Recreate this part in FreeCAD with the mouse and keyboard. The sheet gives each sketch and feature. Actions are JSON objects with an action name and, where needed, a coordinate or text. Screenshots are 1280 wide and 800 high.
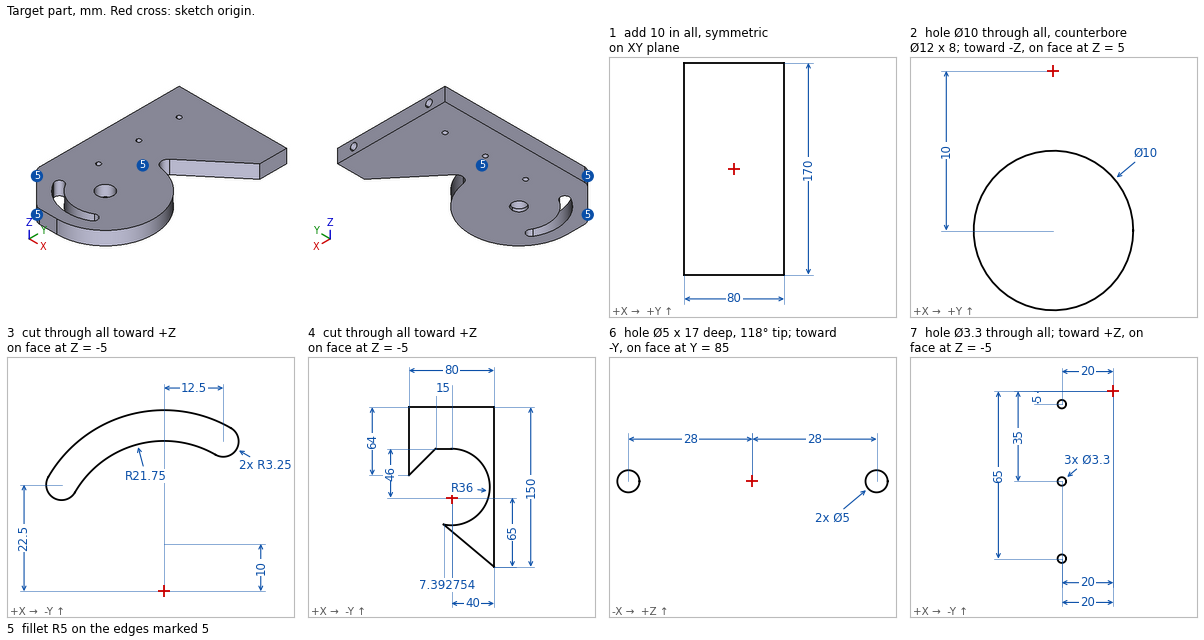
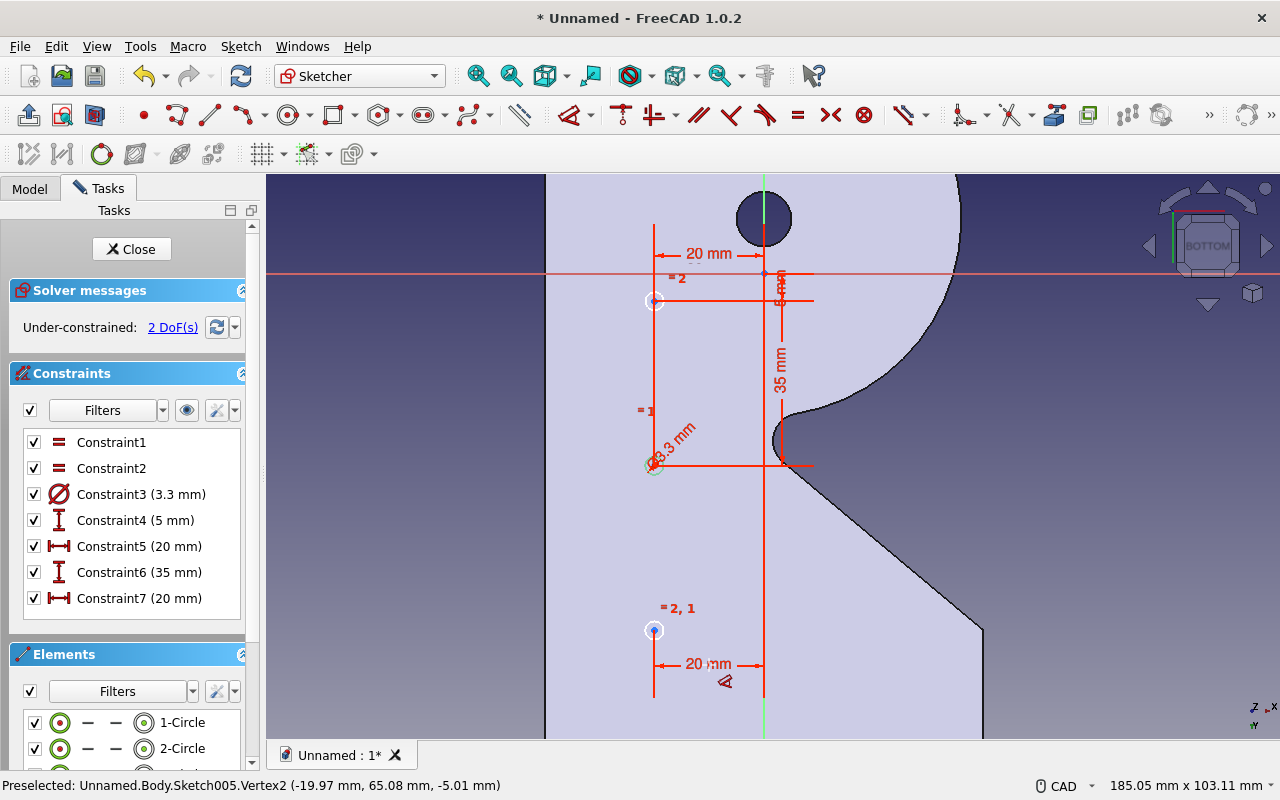
{"action": "left_click", "coordinate": [654, 631]}
{"action": "left_click", "coordinate": [798, 452]}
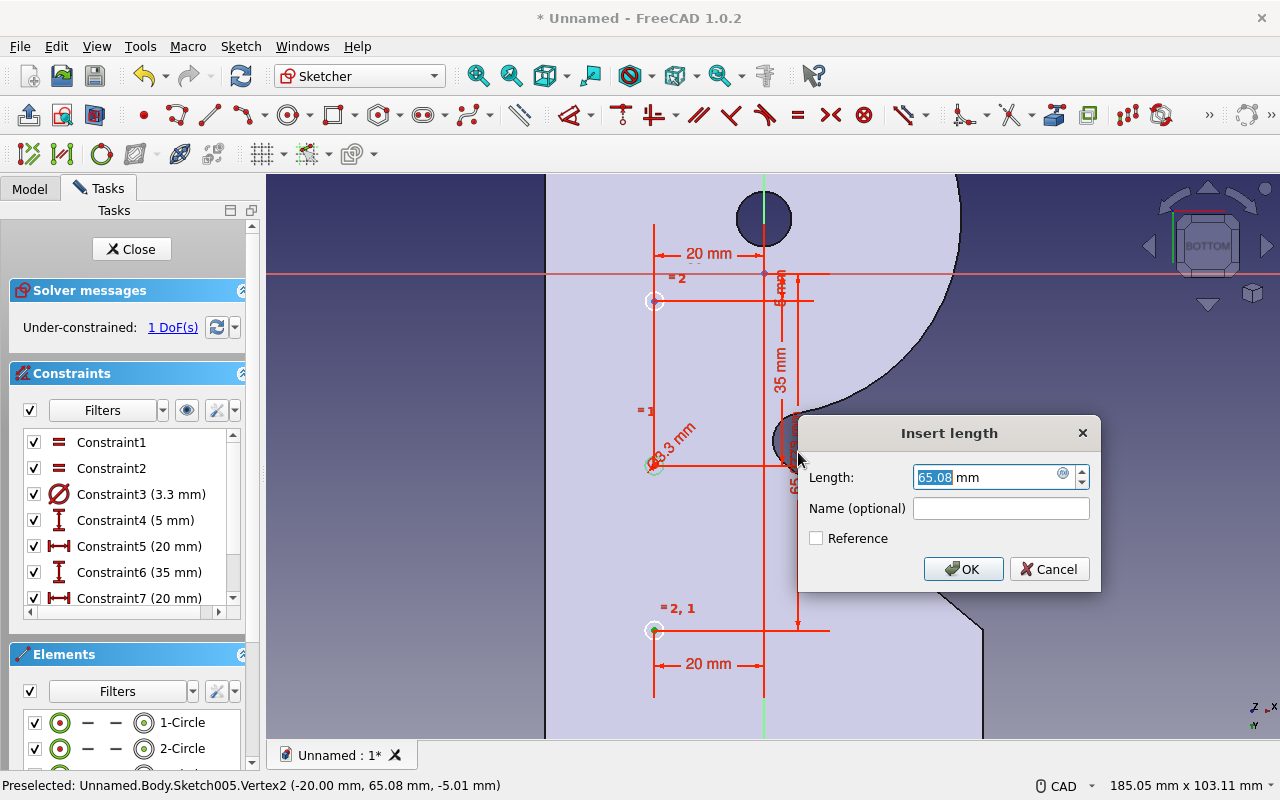
{"action": "type", "text": "65"}
{"action": "key", "text": "Return"}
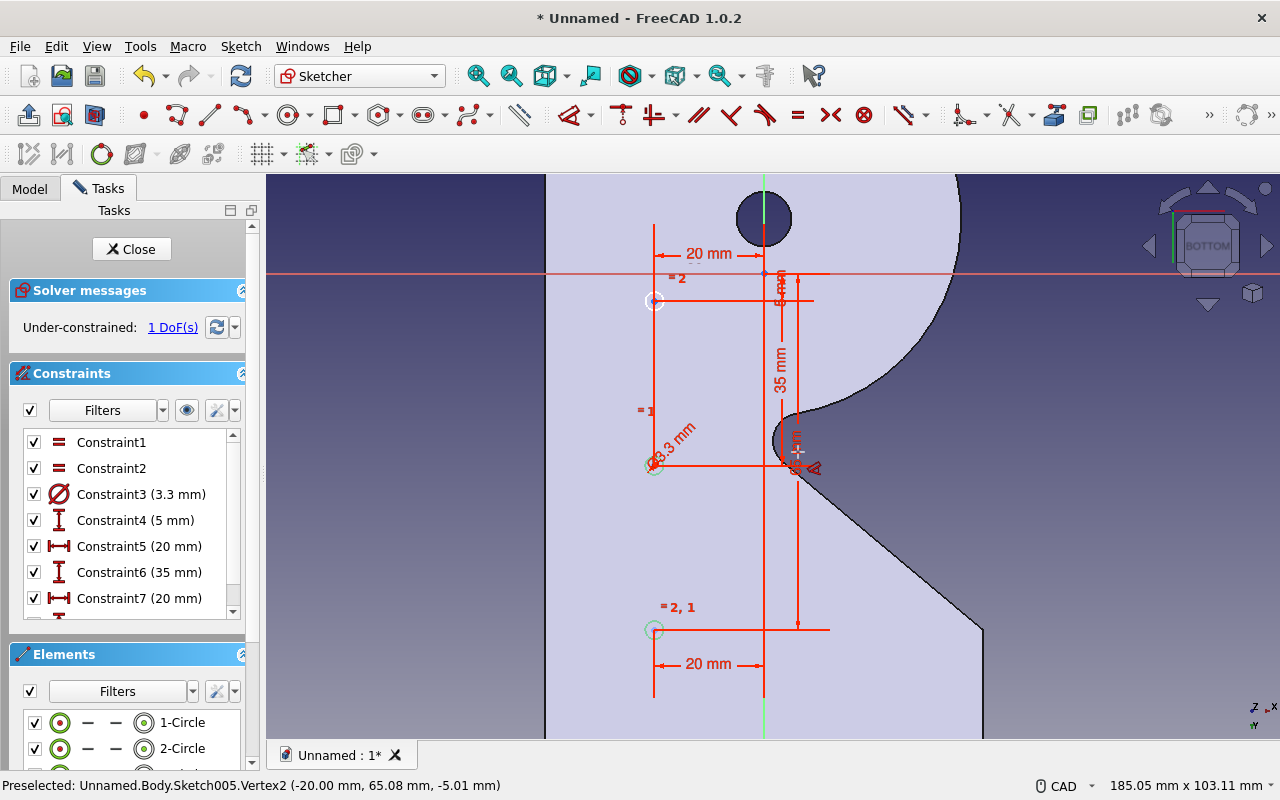
{"action": "left_click", "coordinate": [655, 301]}
{"action": "left_click", "coordinate": [709, 335]}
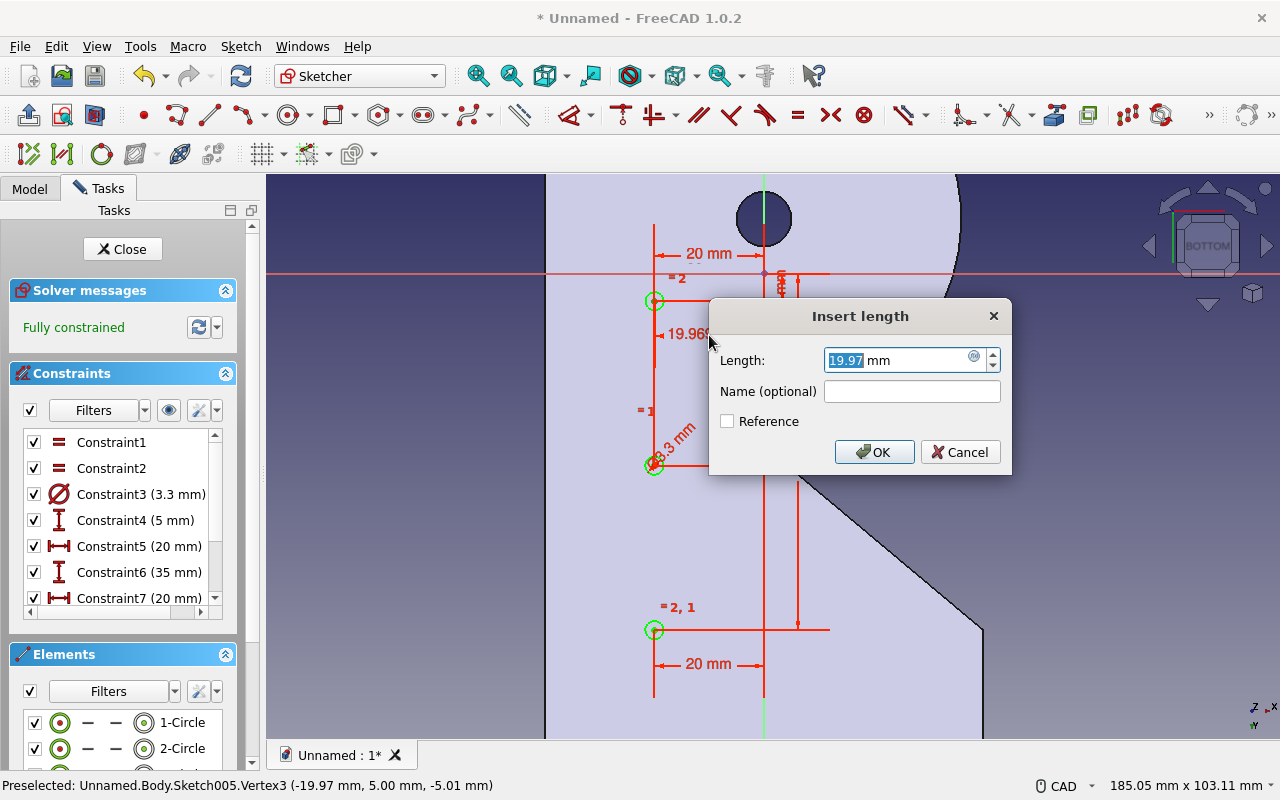
{"action": "type", "text": "20"}
{"action": "key", "text": "Return"}
{"action": "key", "text": "Escape"}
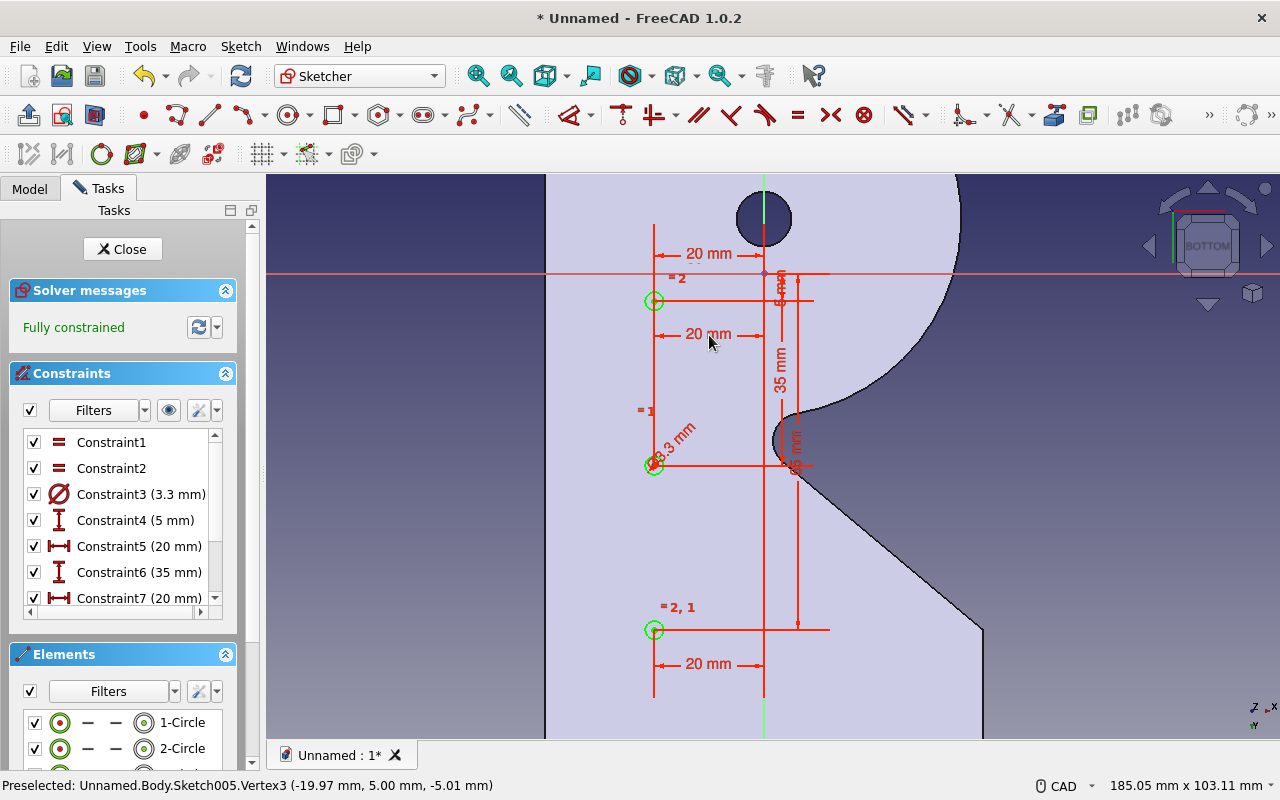
{"action": "left_click", "coordinate": [123, 249]}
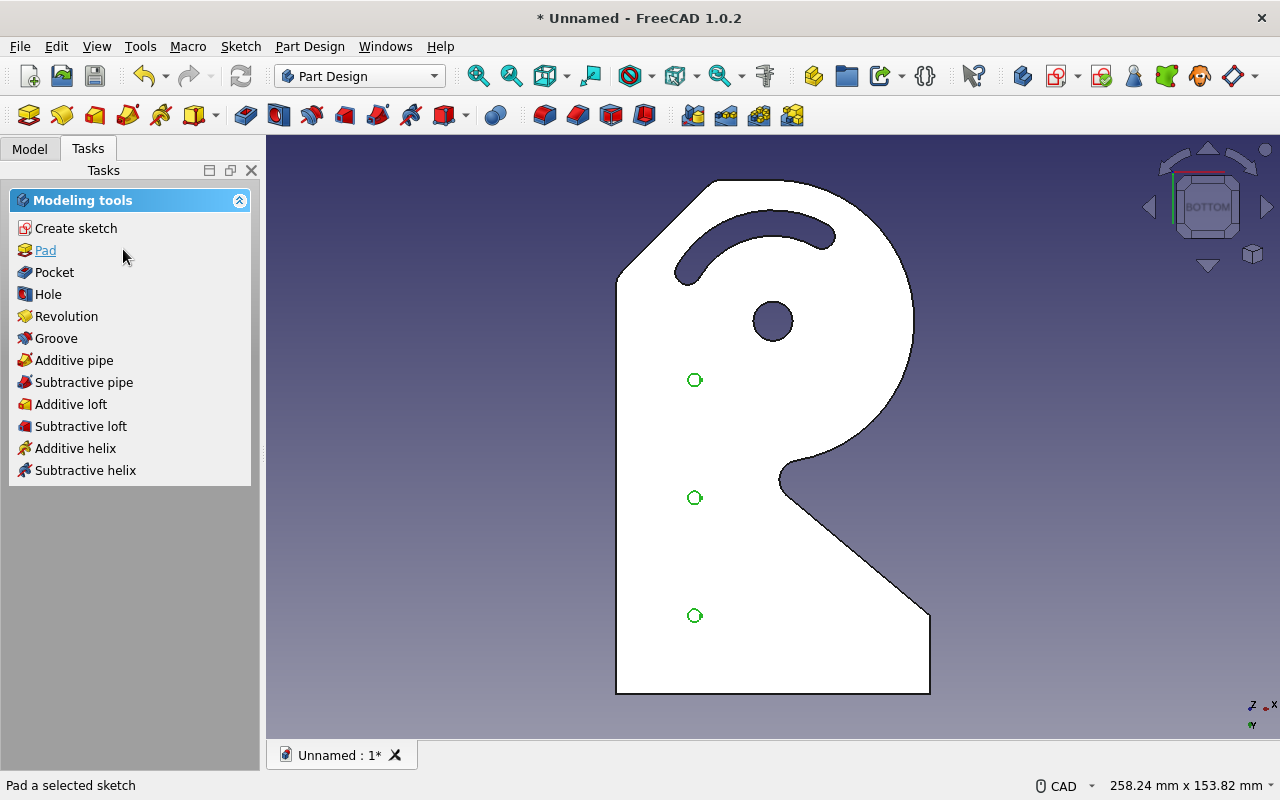
{"action": "left_click", "coordinate": [279, 116]}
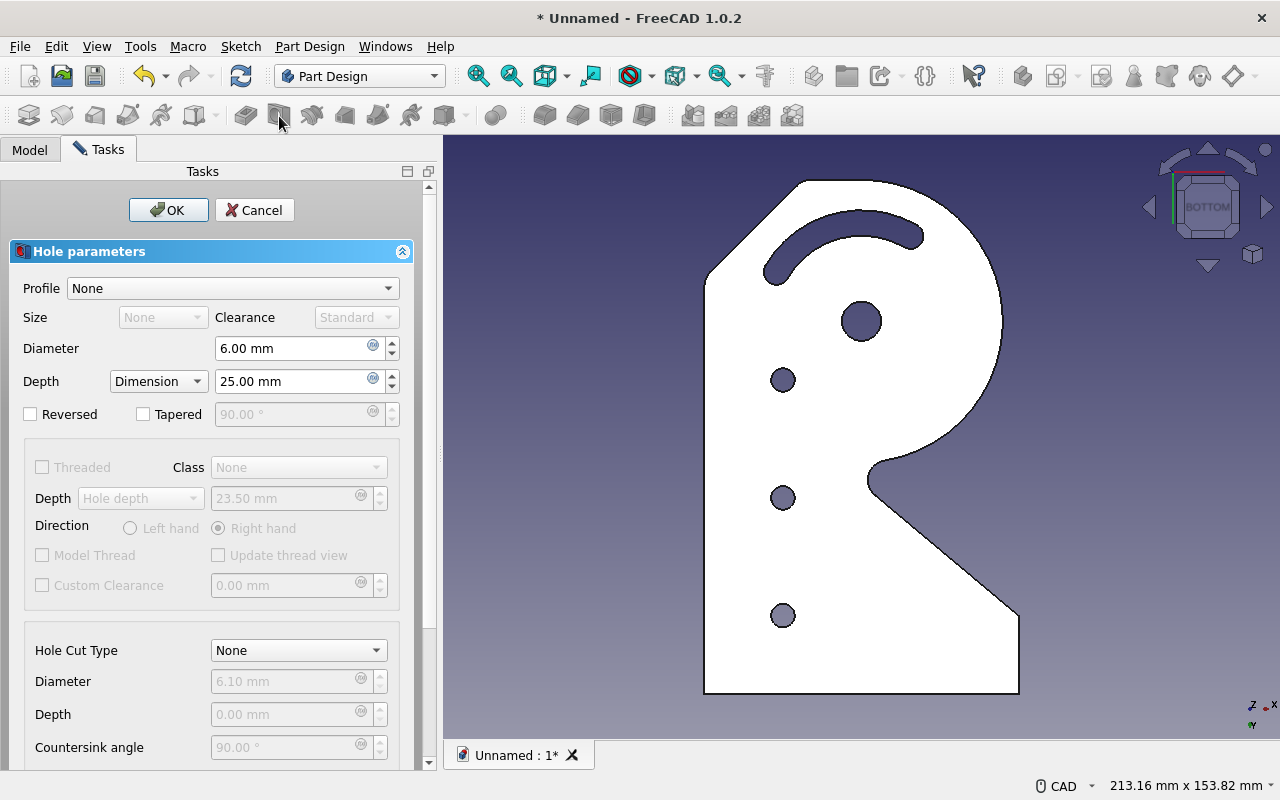
{"action": "triple_click", "coordinate": [300, 348]}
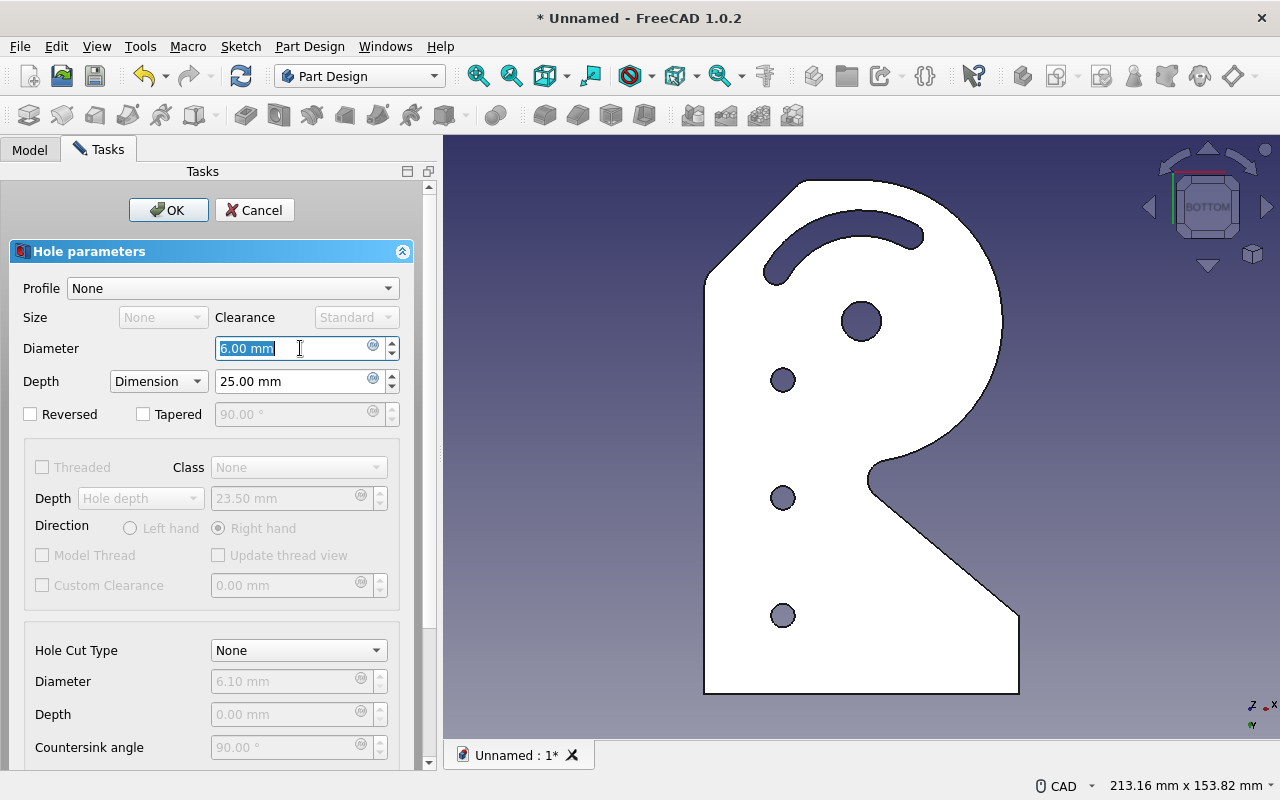
{"action": "type", "text": "3.3"}
{"action": "key", "text": "Tab"}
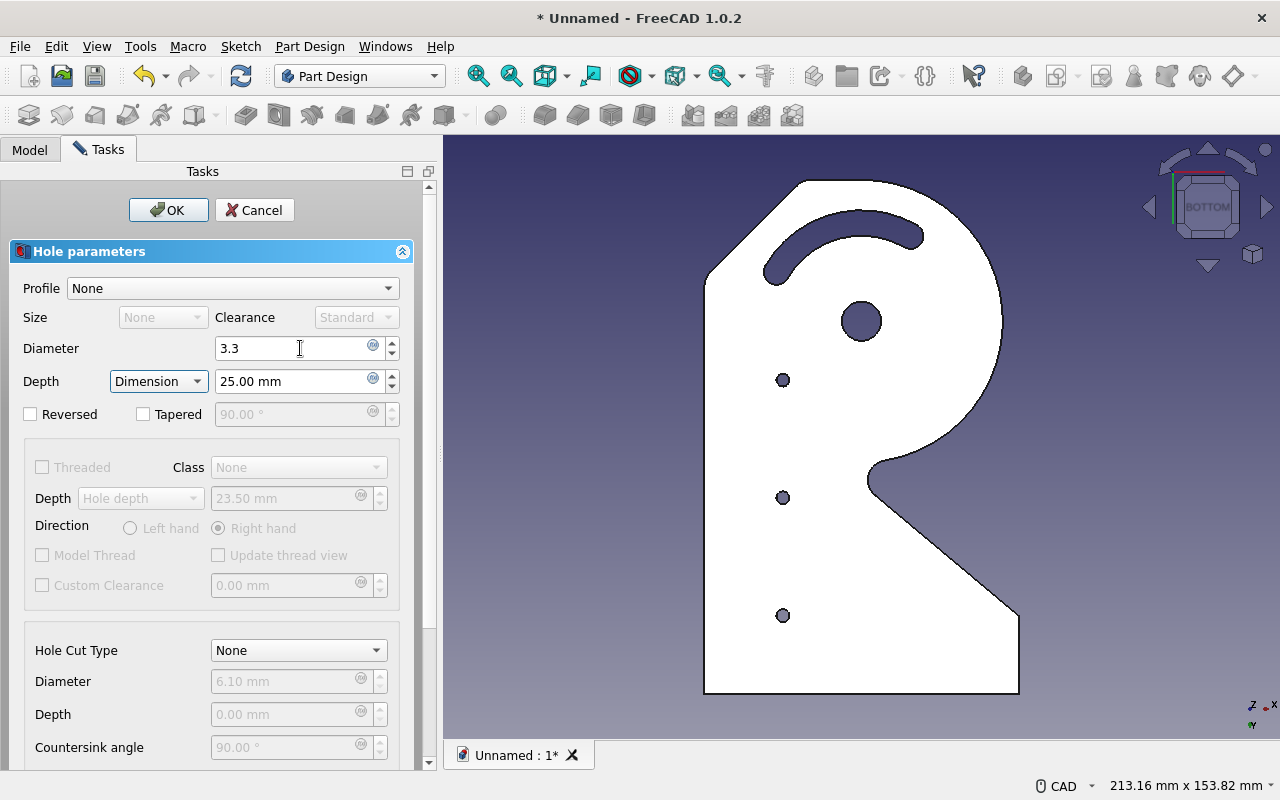
{"action": "left_click", "coordinate": [160, 382]}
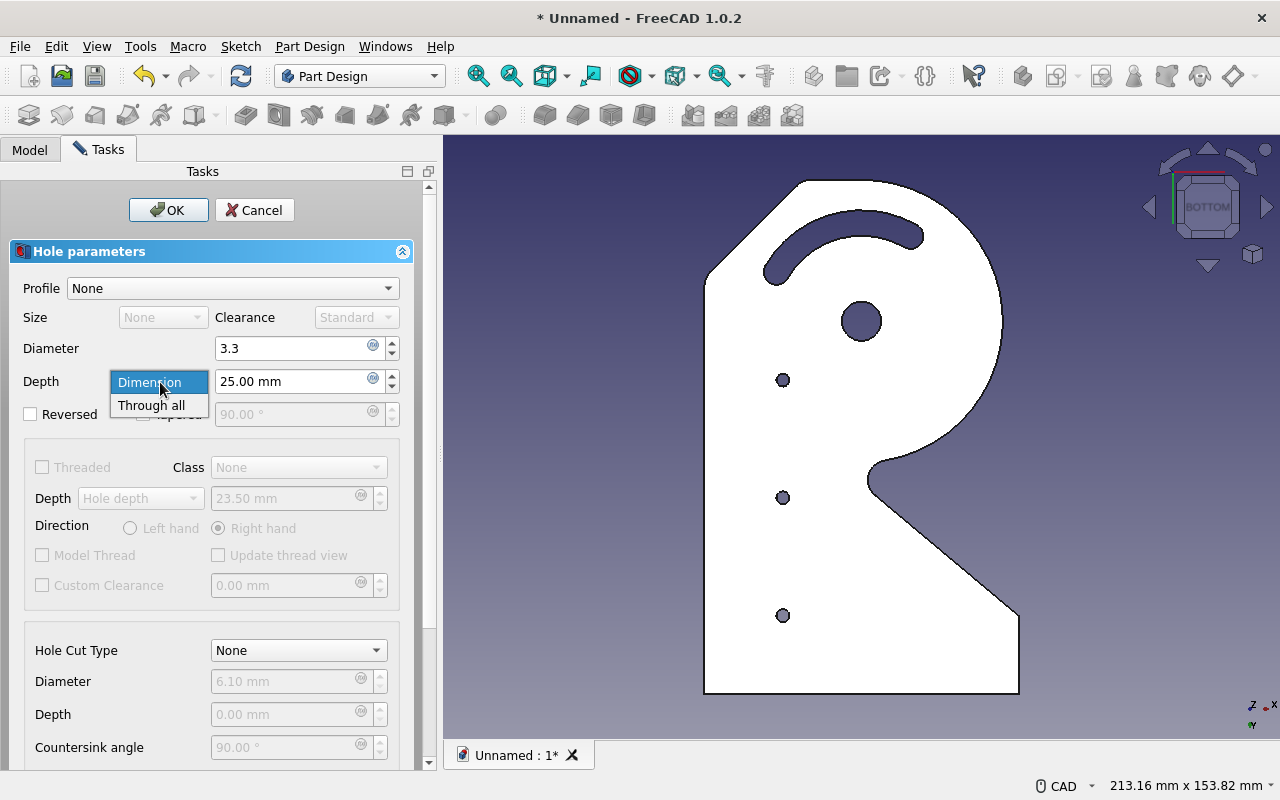
{"action": "left_click", "coordinate": [158, 406]}